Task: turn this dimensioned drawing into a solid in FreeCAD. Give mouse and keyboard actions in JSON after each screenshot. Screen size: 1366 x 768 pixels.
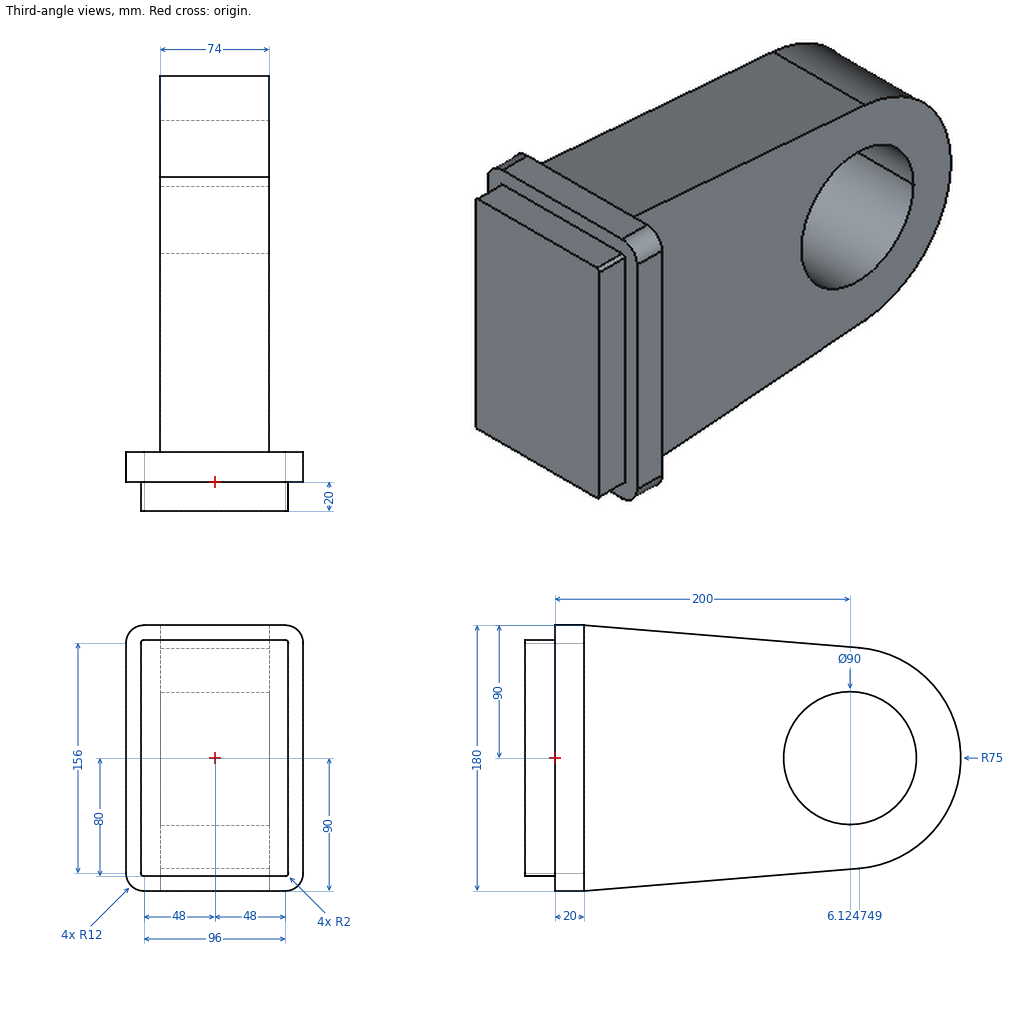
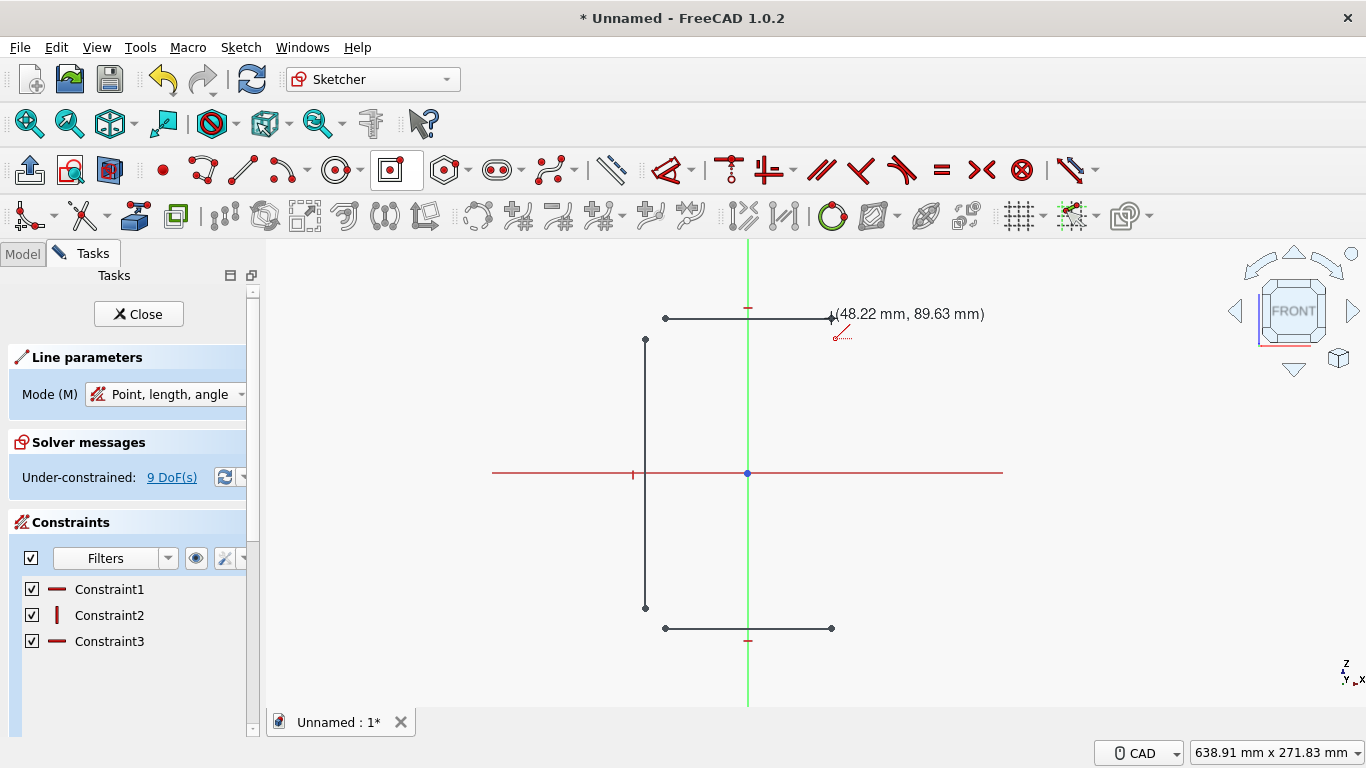
{"action": "left_click", "coordinate": [851, 339]}
{"action": "left_click", "coordinate": [851, 608]}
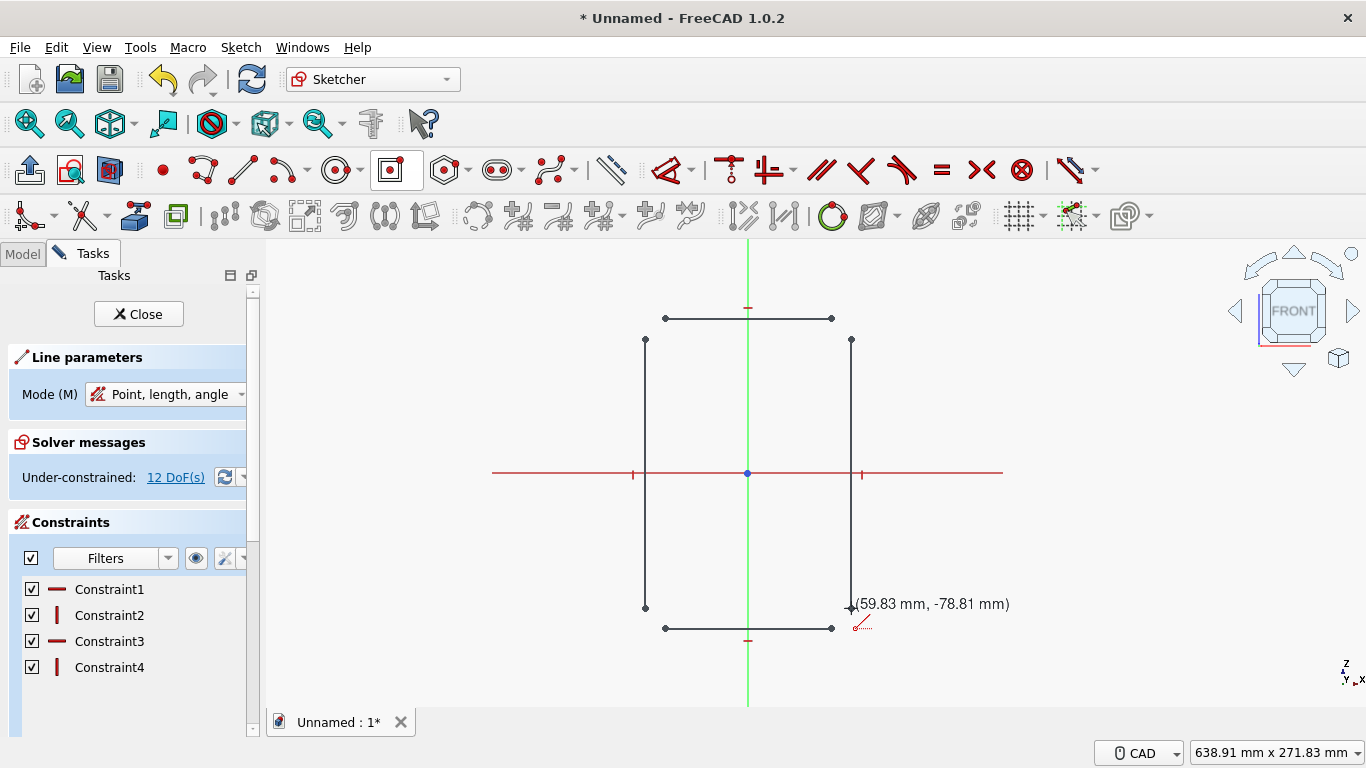
{"action": "key", "text": "g 3 a"}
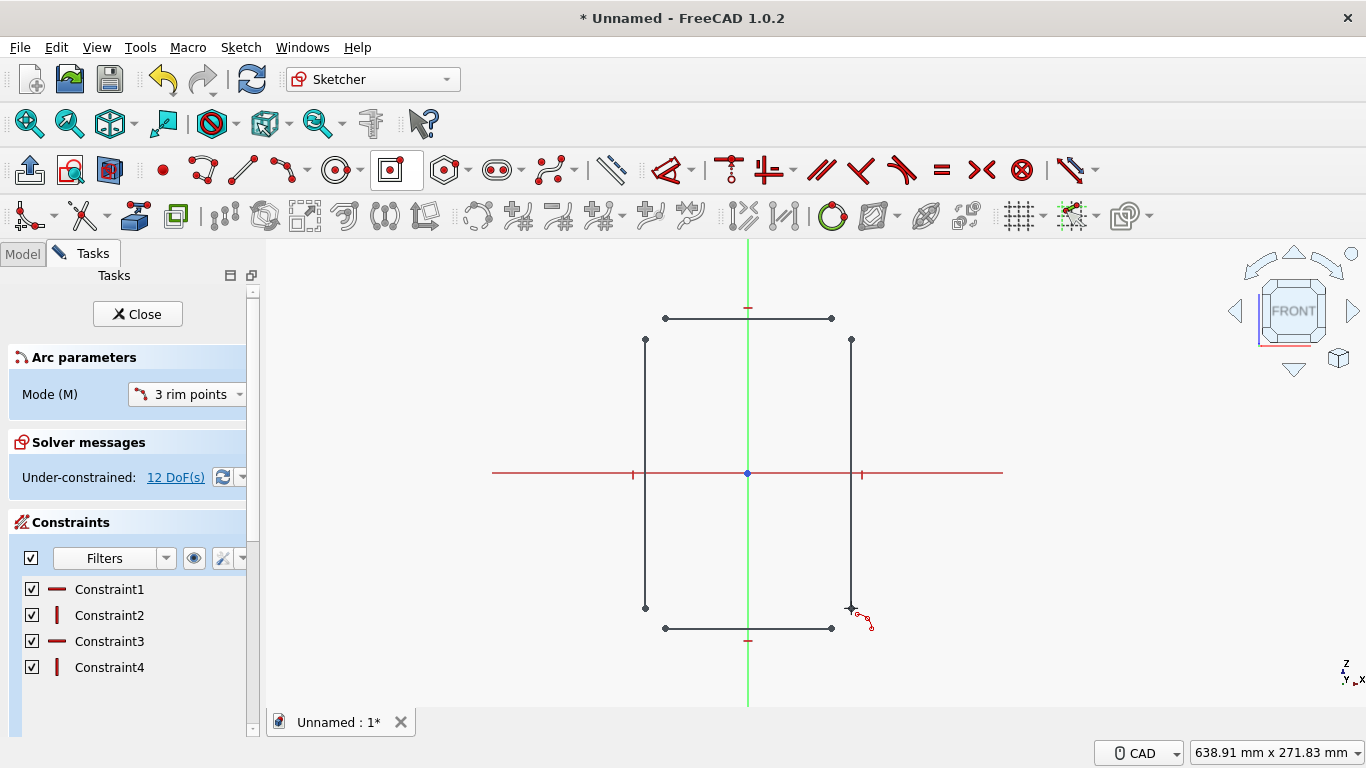
{"action": "left_click", "coordinate": [665, 629]}
{"action": "left_click", "coordinate": [645, 609]}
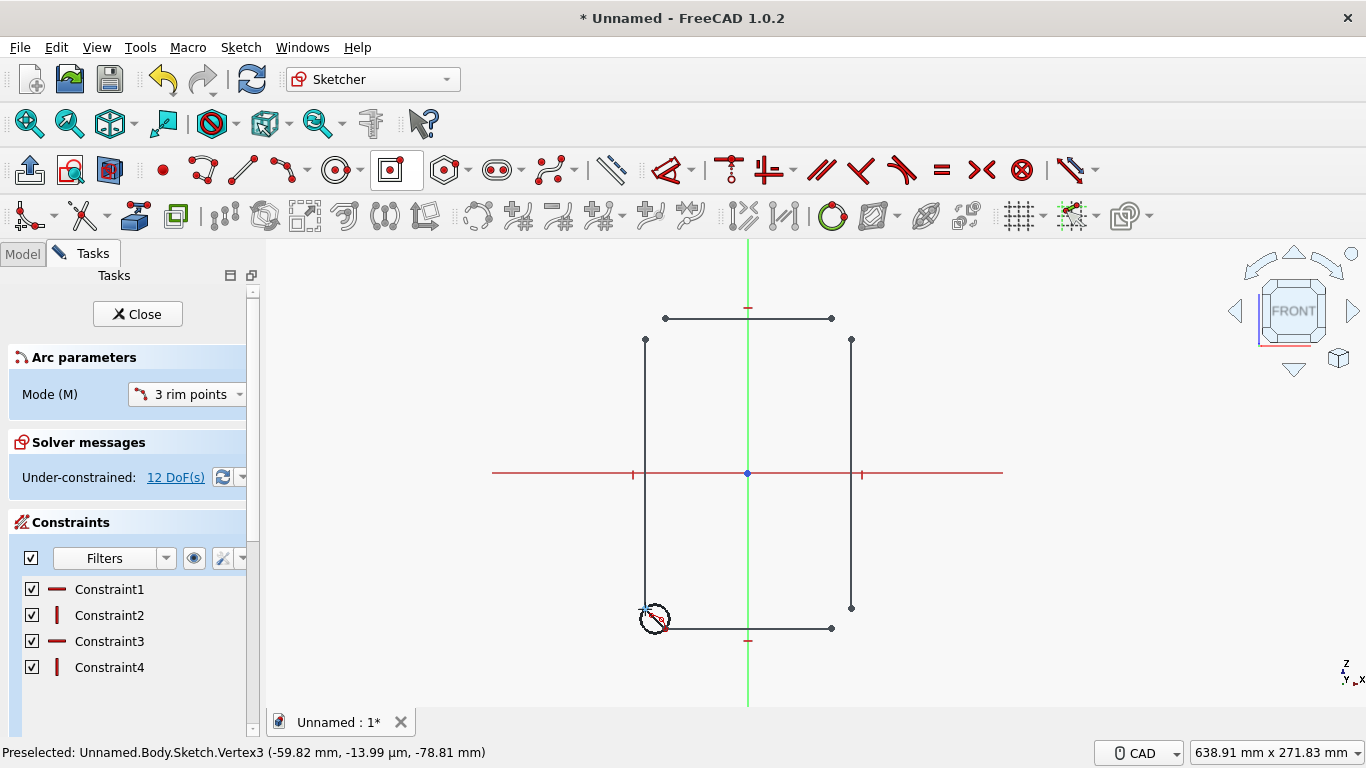
{"action": "scroll", "coordinate": [651, 622], "scroll_direction": "up", "scroll_amount": 5}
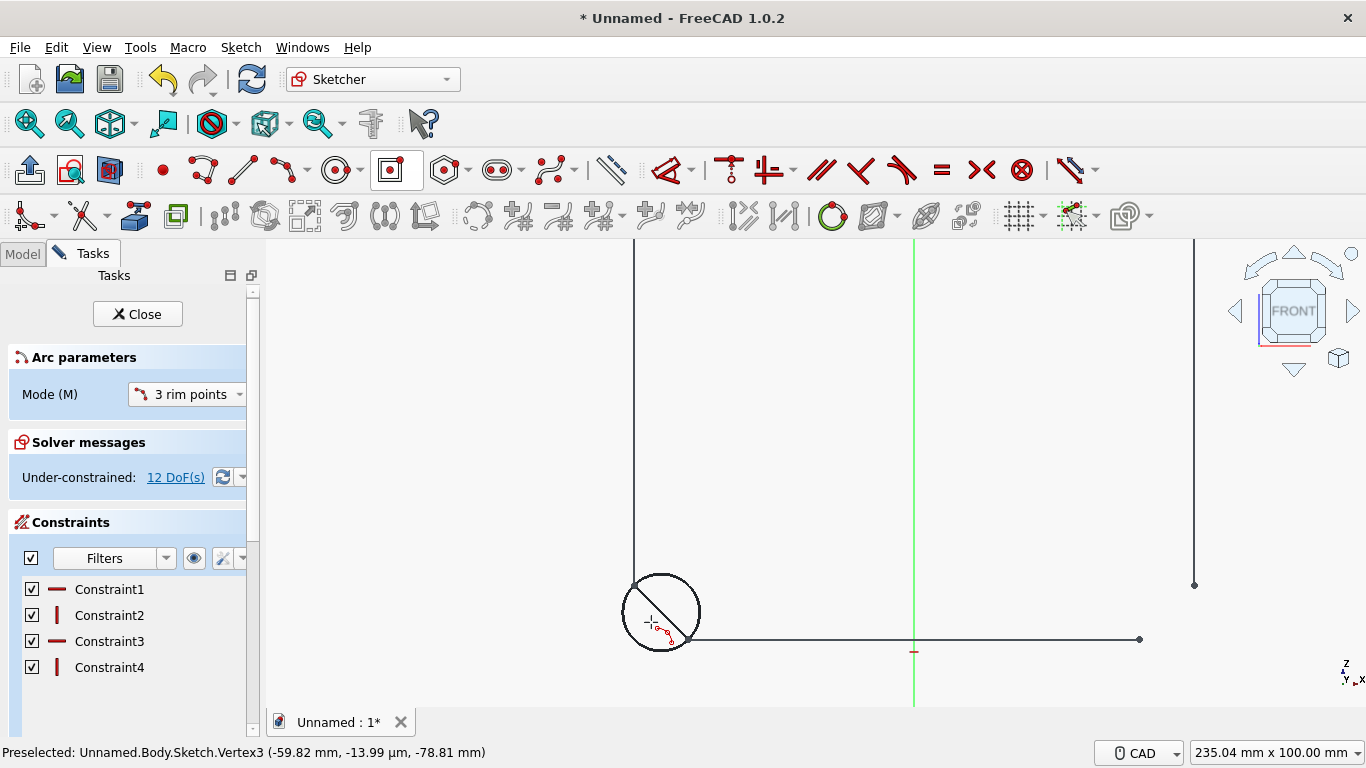
{"action": "left_click", "coordinate": [650, 621]}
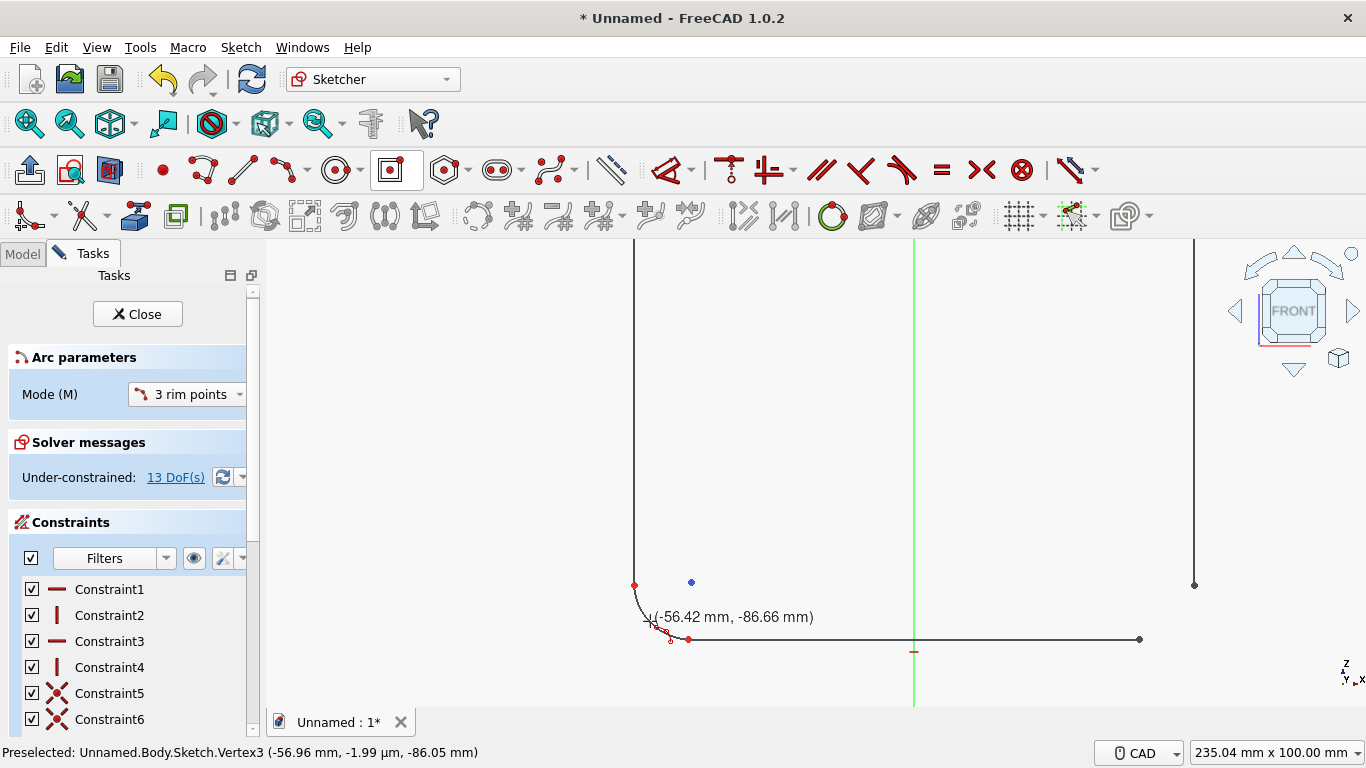
{"action": "scroll", "coordinate": [651, 622], "scroll_direction": "down", "scroll_amount": 5}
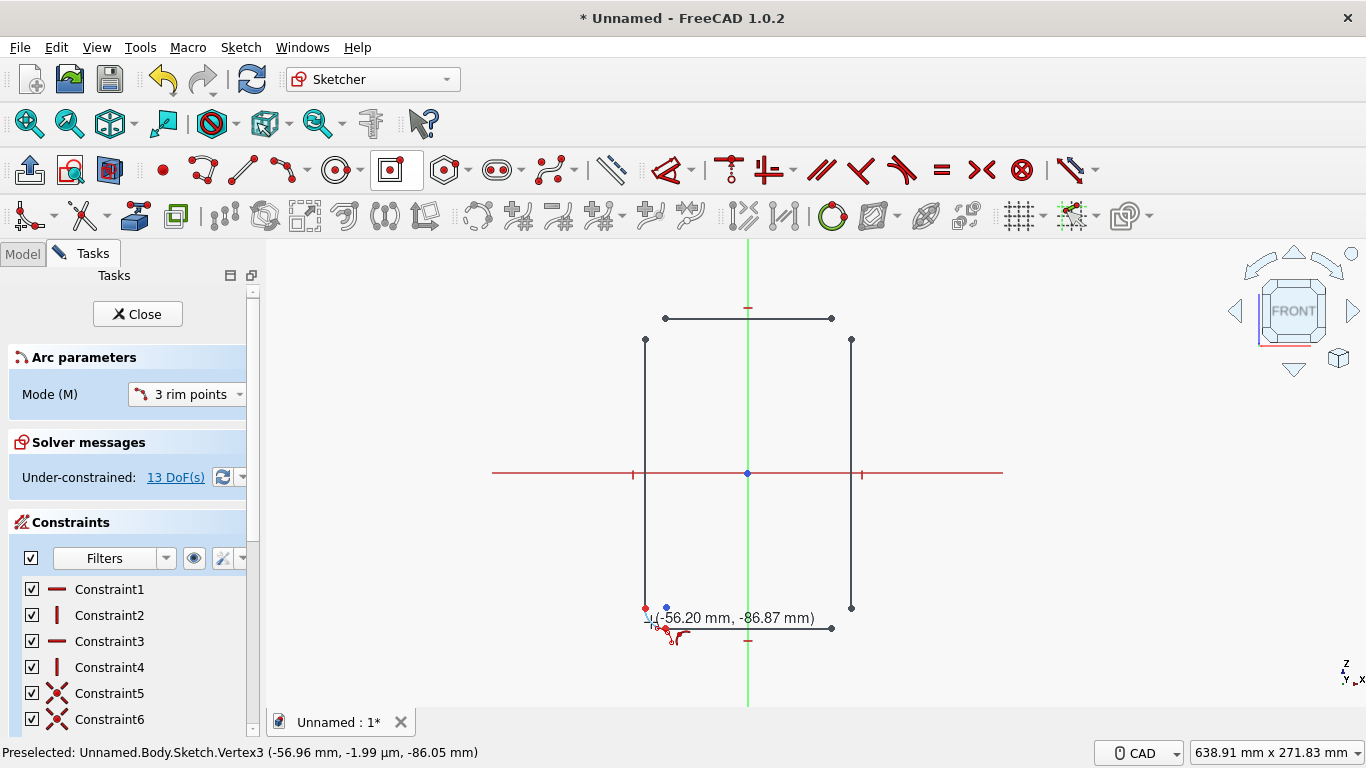
{"action": "left_click", "coordinate": [645, 340]}
{"action": "left_click", "coordinate": [665, 319]}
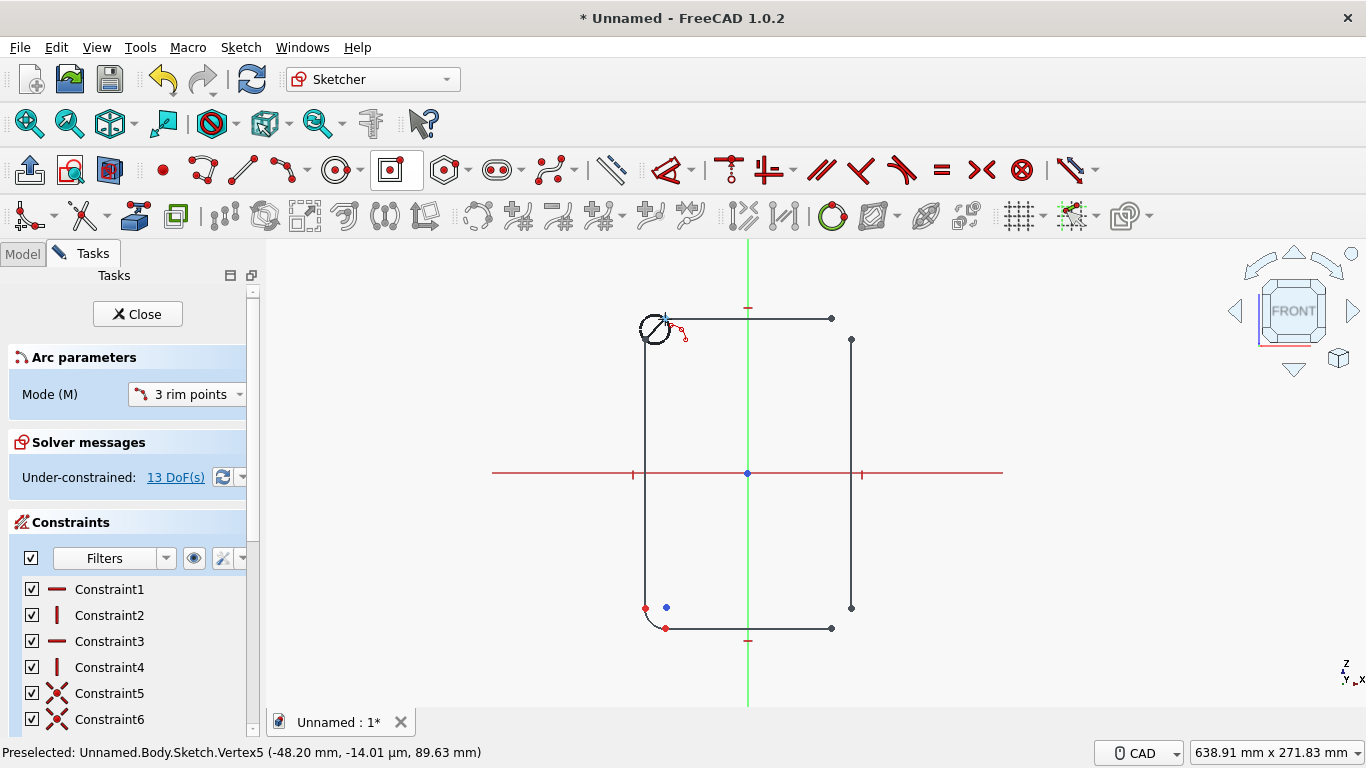
{"action": "scroll", "coordinate": [651, 324], "scroll_direction": "up", "scroll_amount": 5}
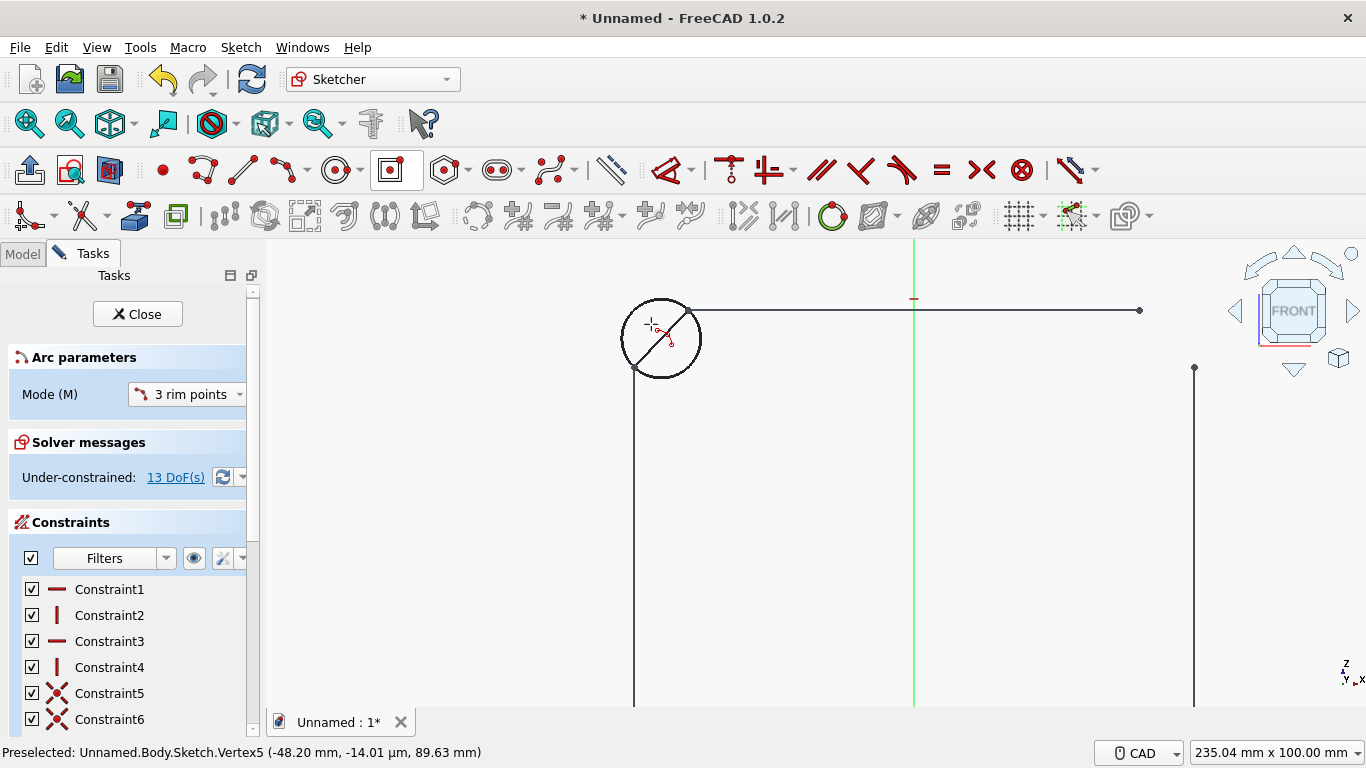
{"action": "left_click", "coordinate": [650, 325]}